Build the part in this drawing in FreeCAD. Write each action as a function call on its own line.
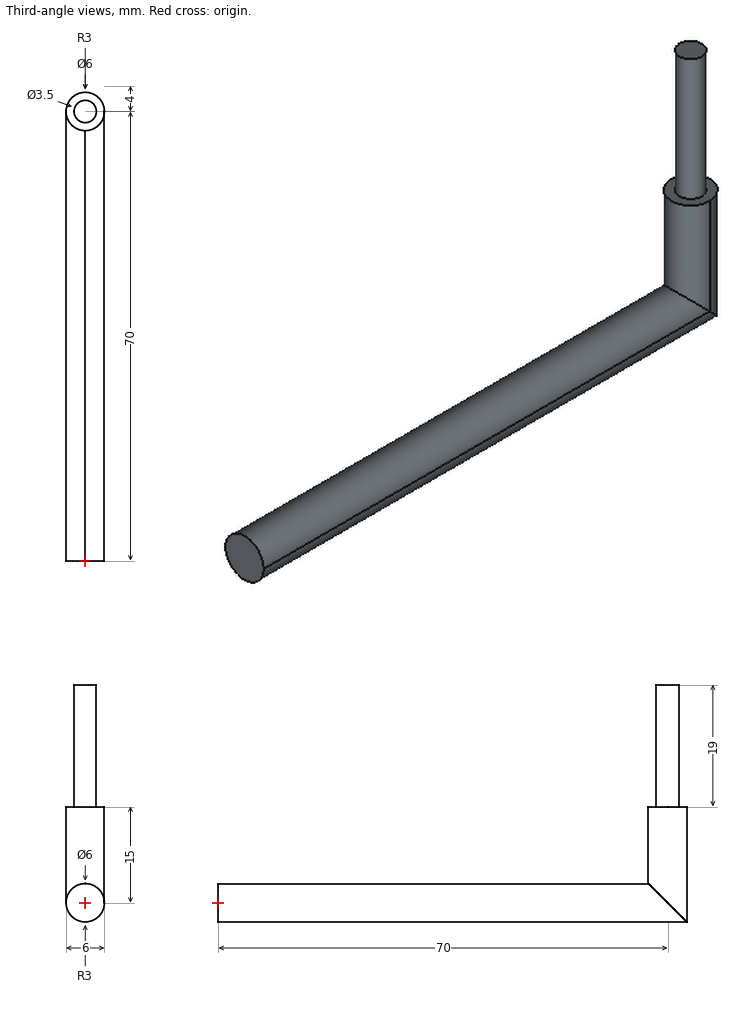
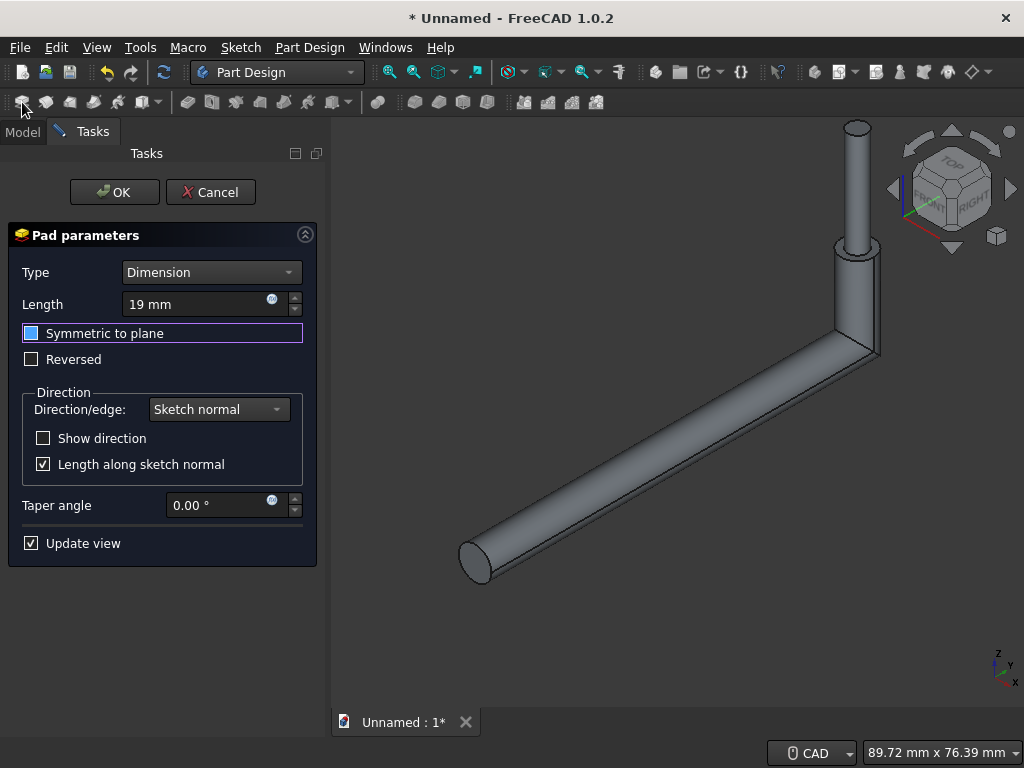
click(115, 192)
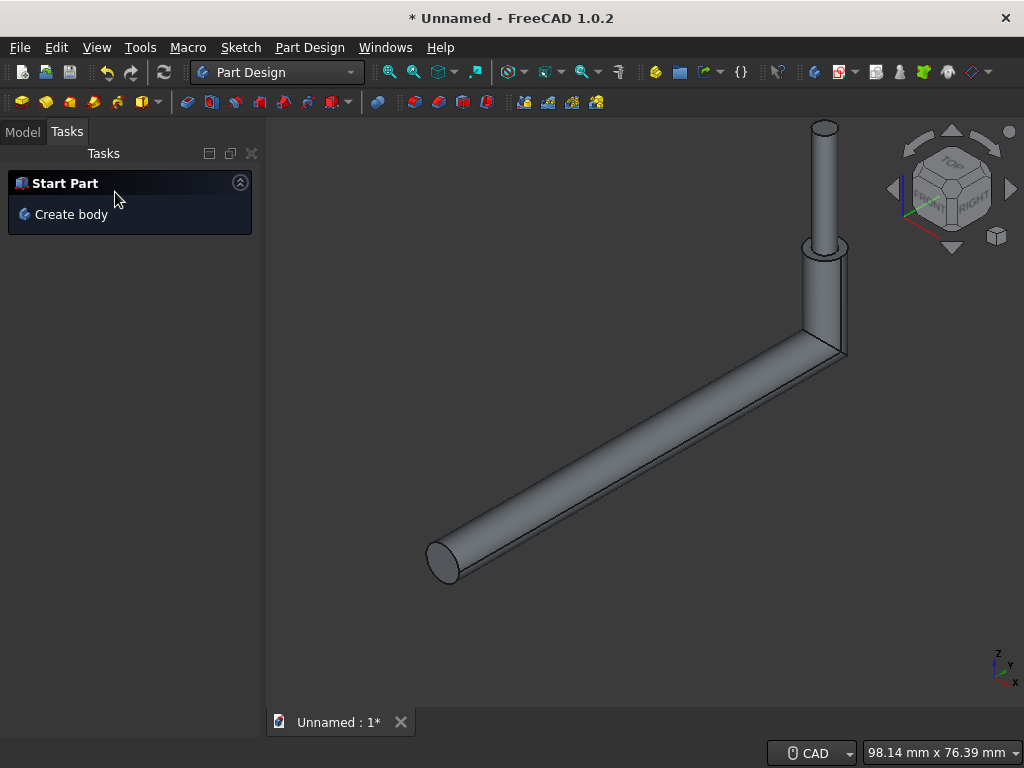
key(v)
key(f)